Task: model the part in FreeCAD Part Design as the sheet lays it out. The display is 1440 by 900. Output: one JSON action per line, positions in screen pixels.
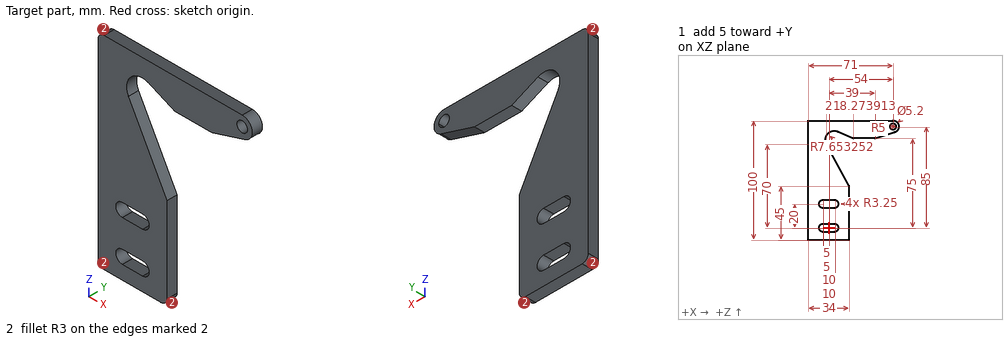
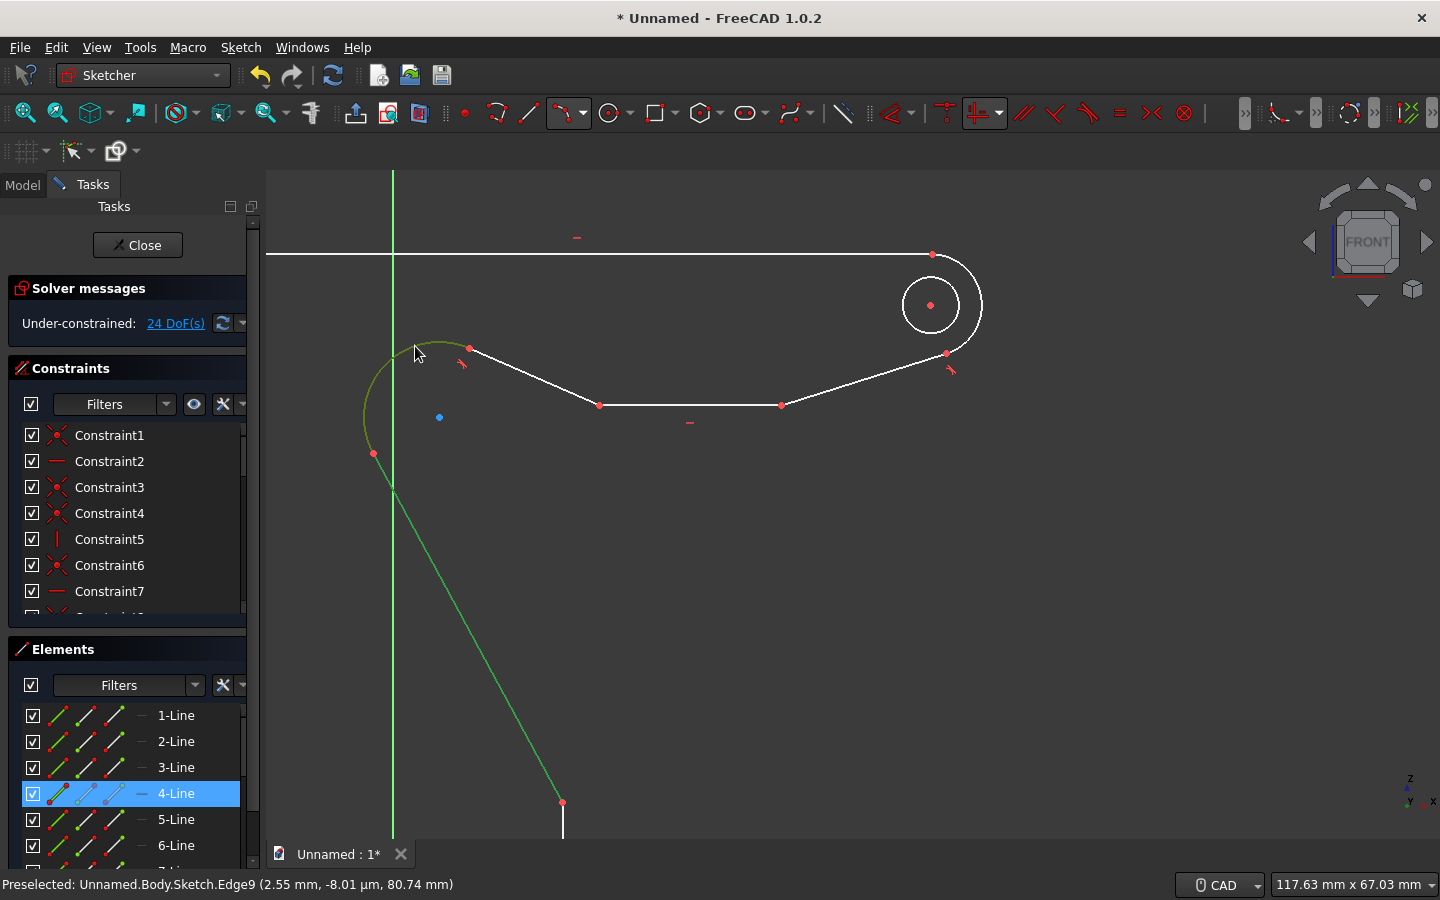
{"action": "left_click", "coordinate": [1088, 114]}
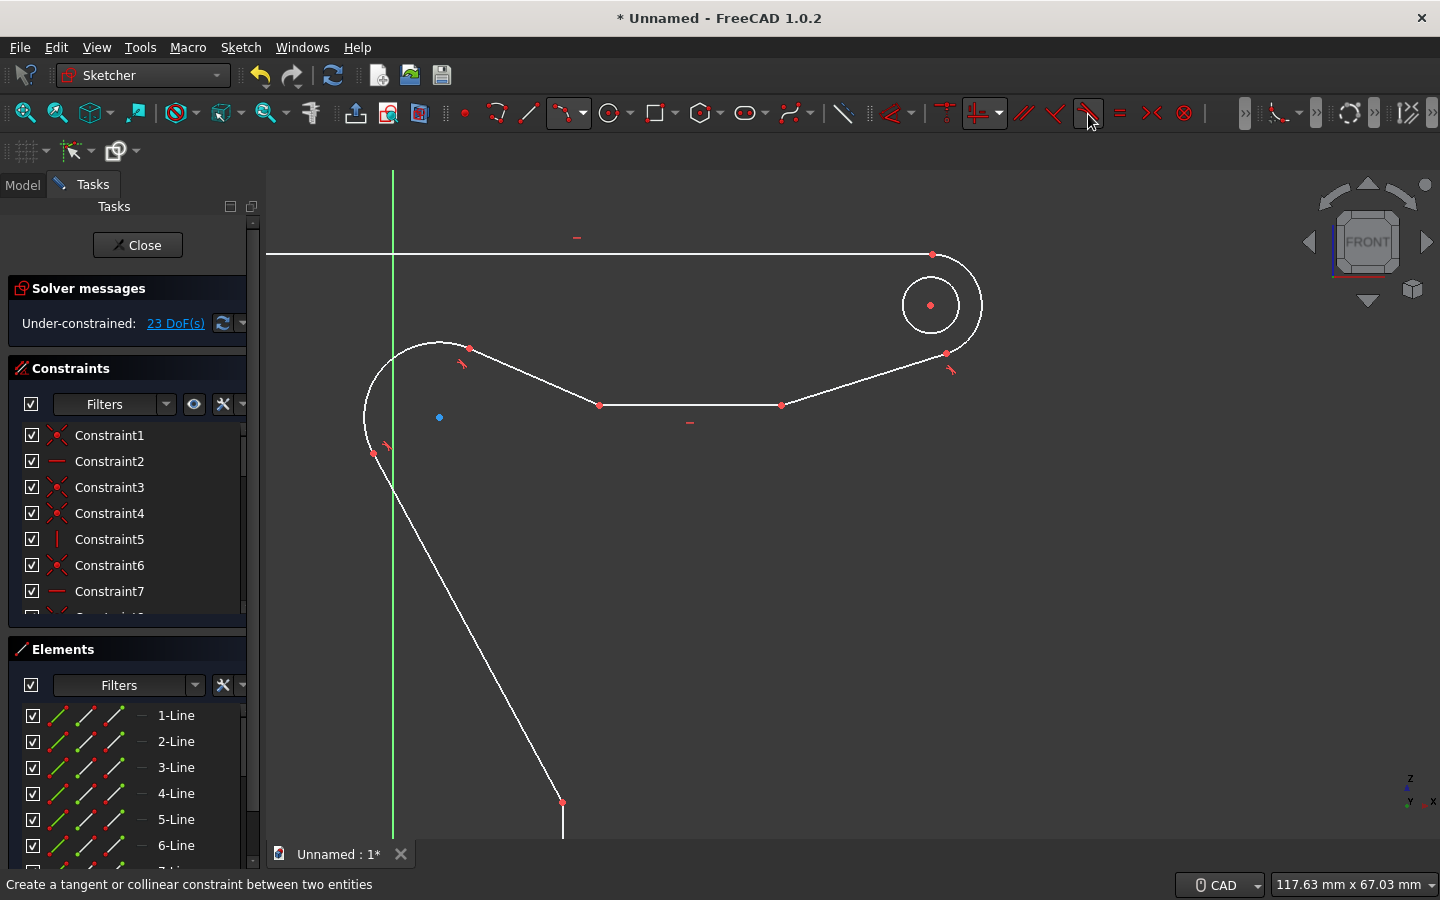
{"action": "left_click", "coordinate": [435, 254]}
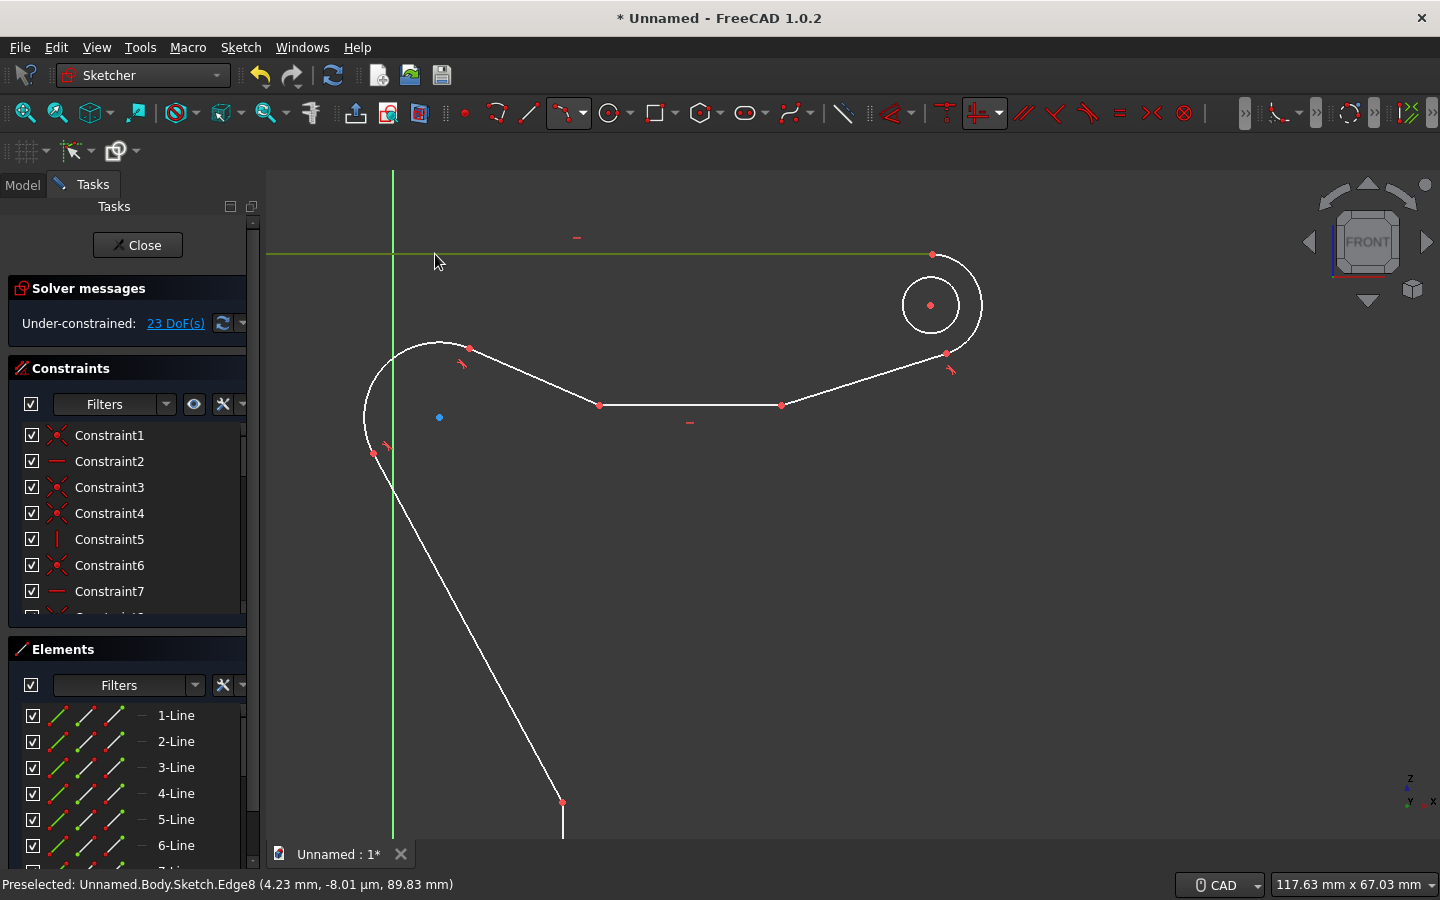
{"action": "left_click", "coordinate": [977, 326]}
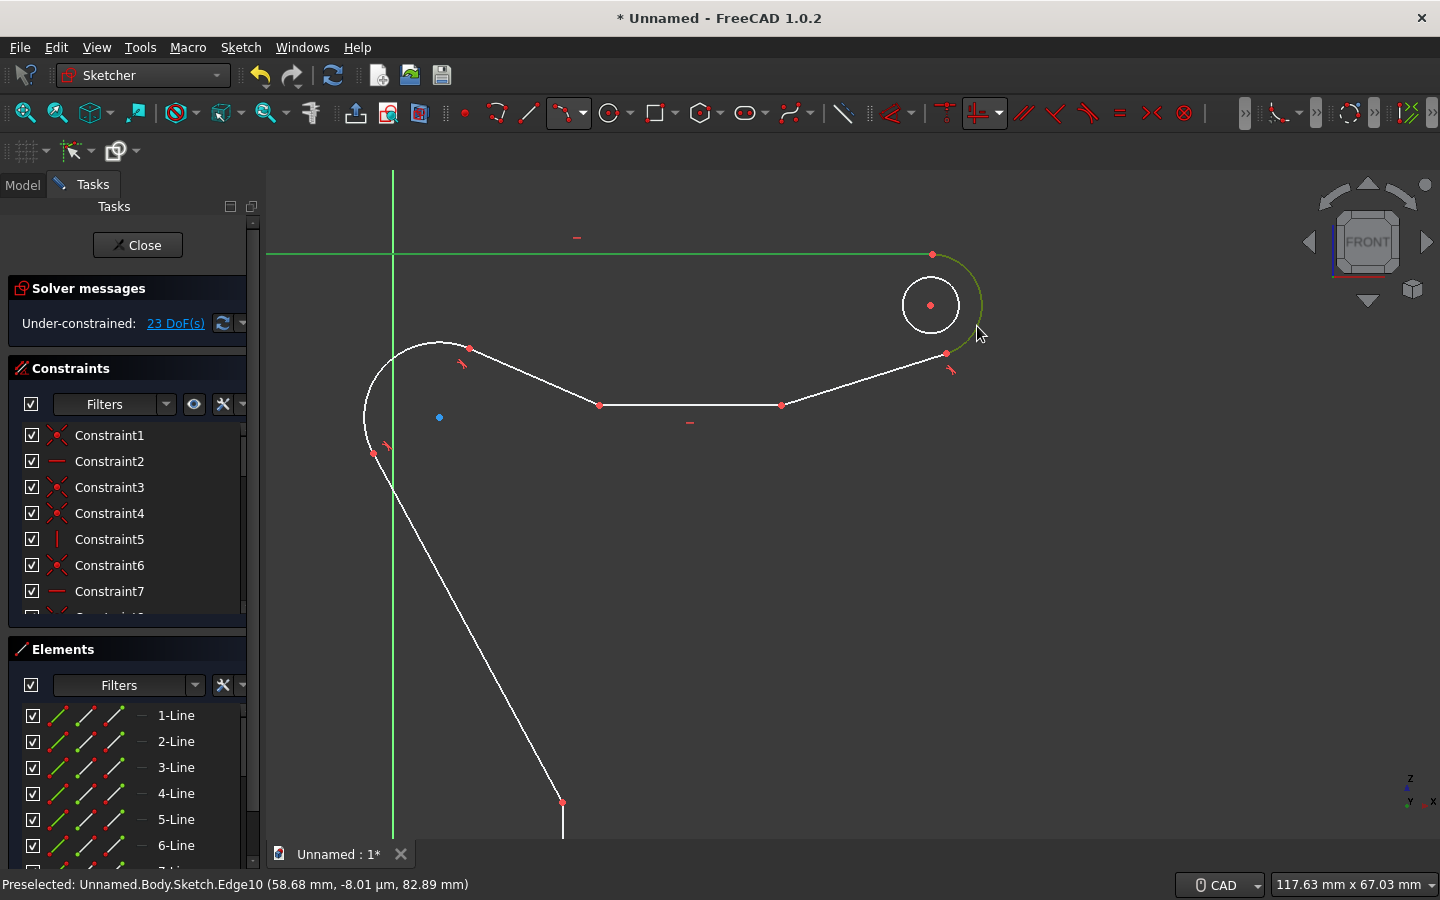
{"action": "left_click", "coordinate": [1088, 114]}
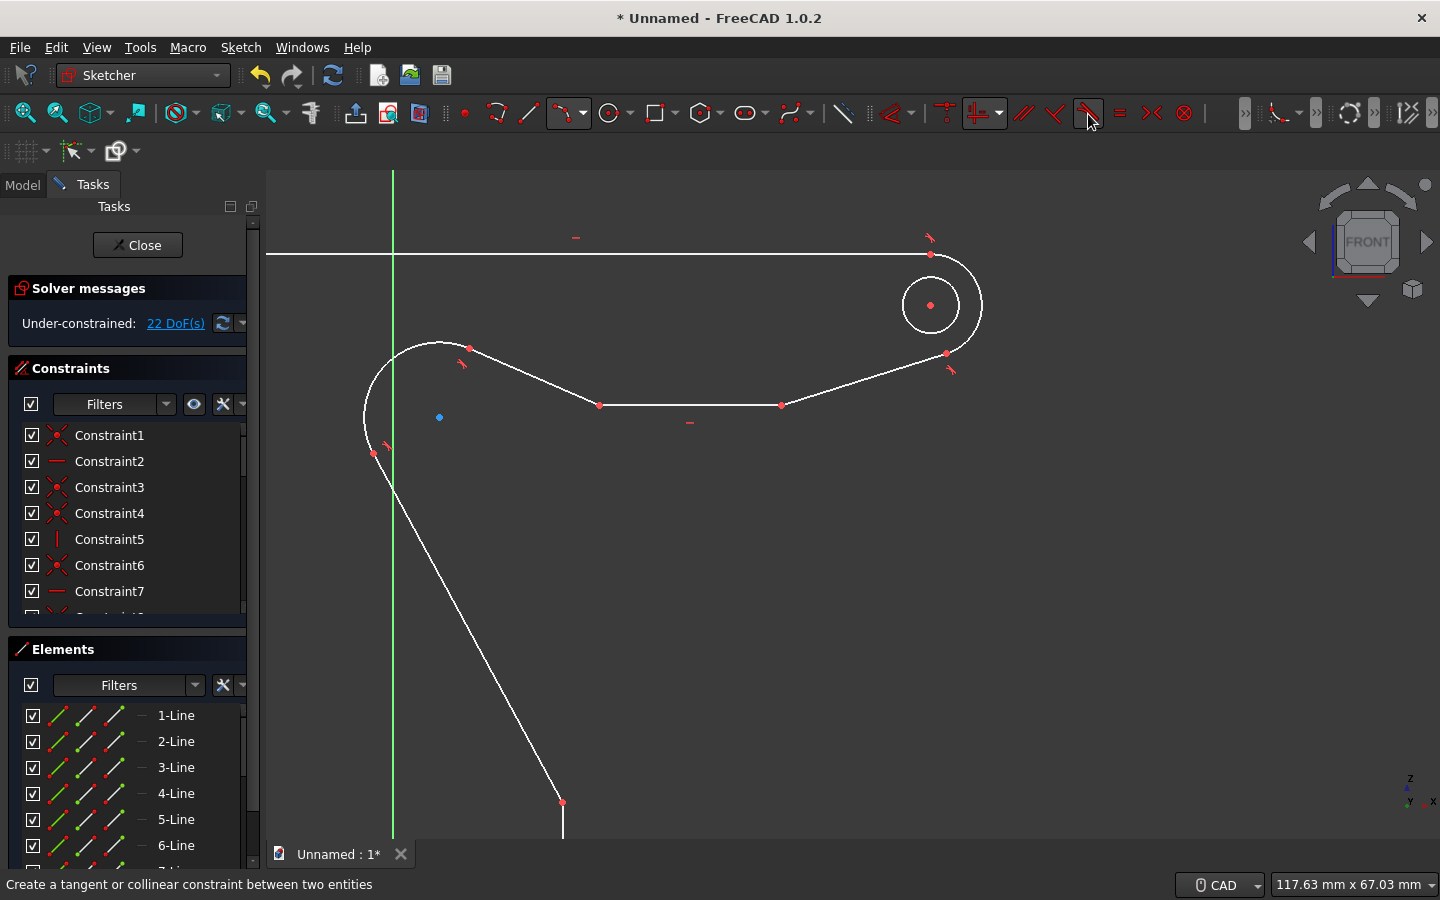
{"action": "scroll", "coordinate": [933, 303], "scroll_direction": "down", "scroll_amount": 4}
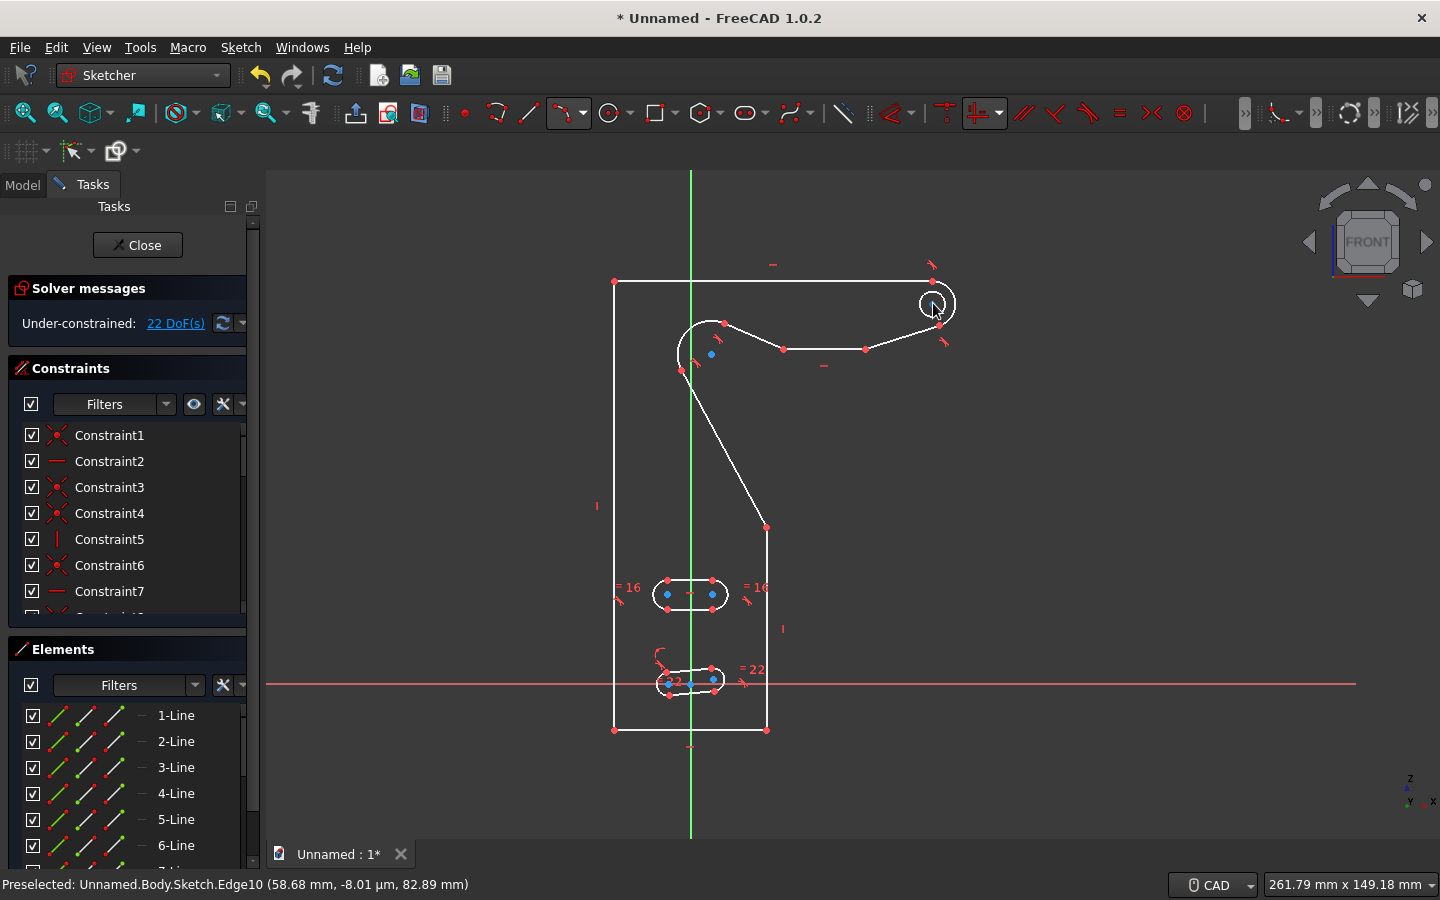
{"action": "scroll", "coordinate": [680, 671], "scroll_direction": "up", "scroll_amount": 2}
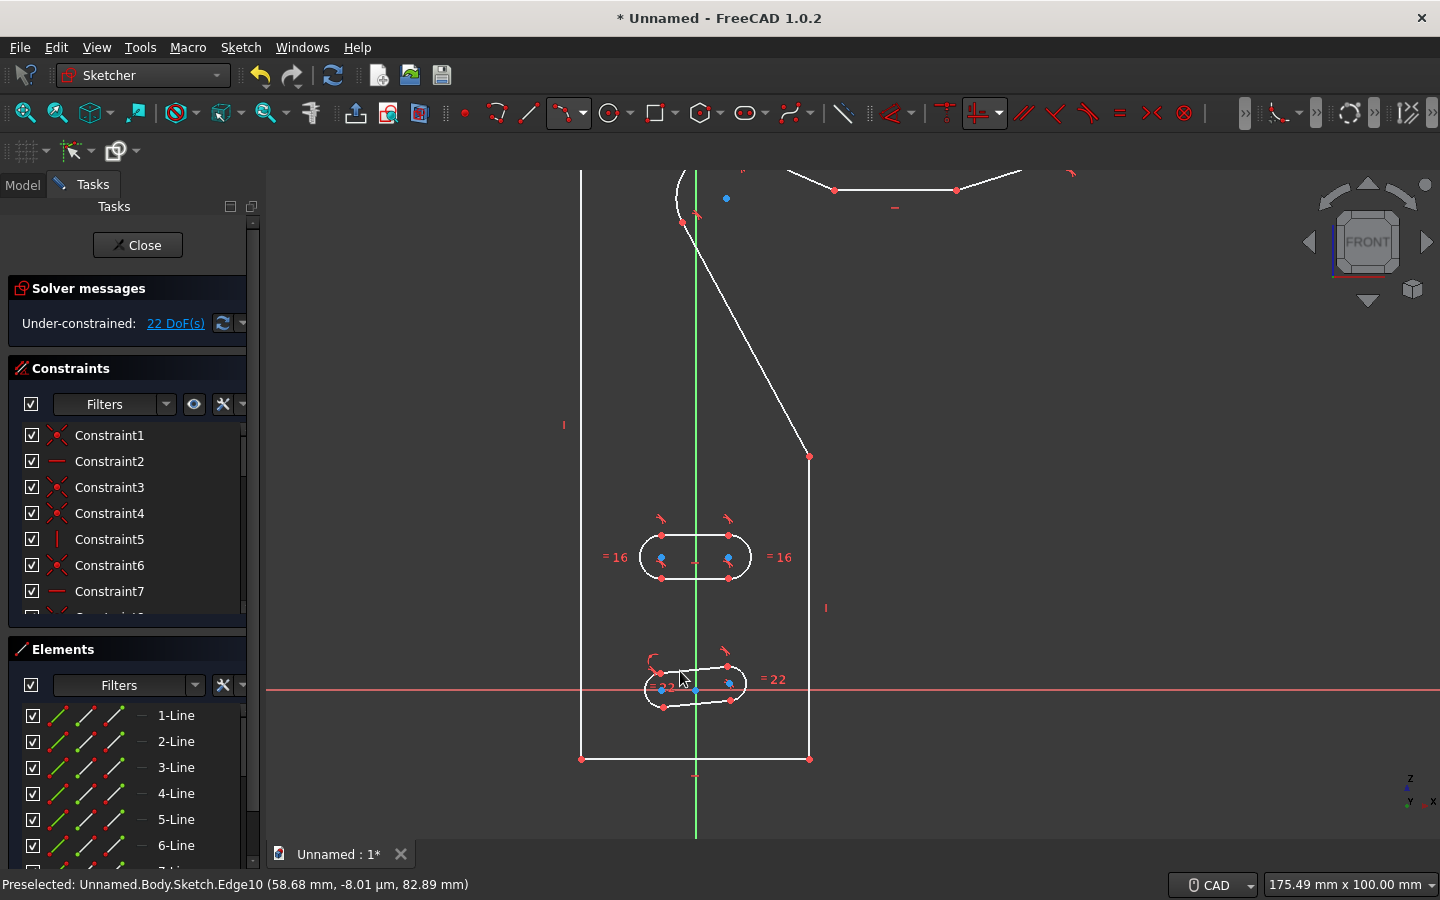
{"action": "left_click", "coordinate": [681, 671]}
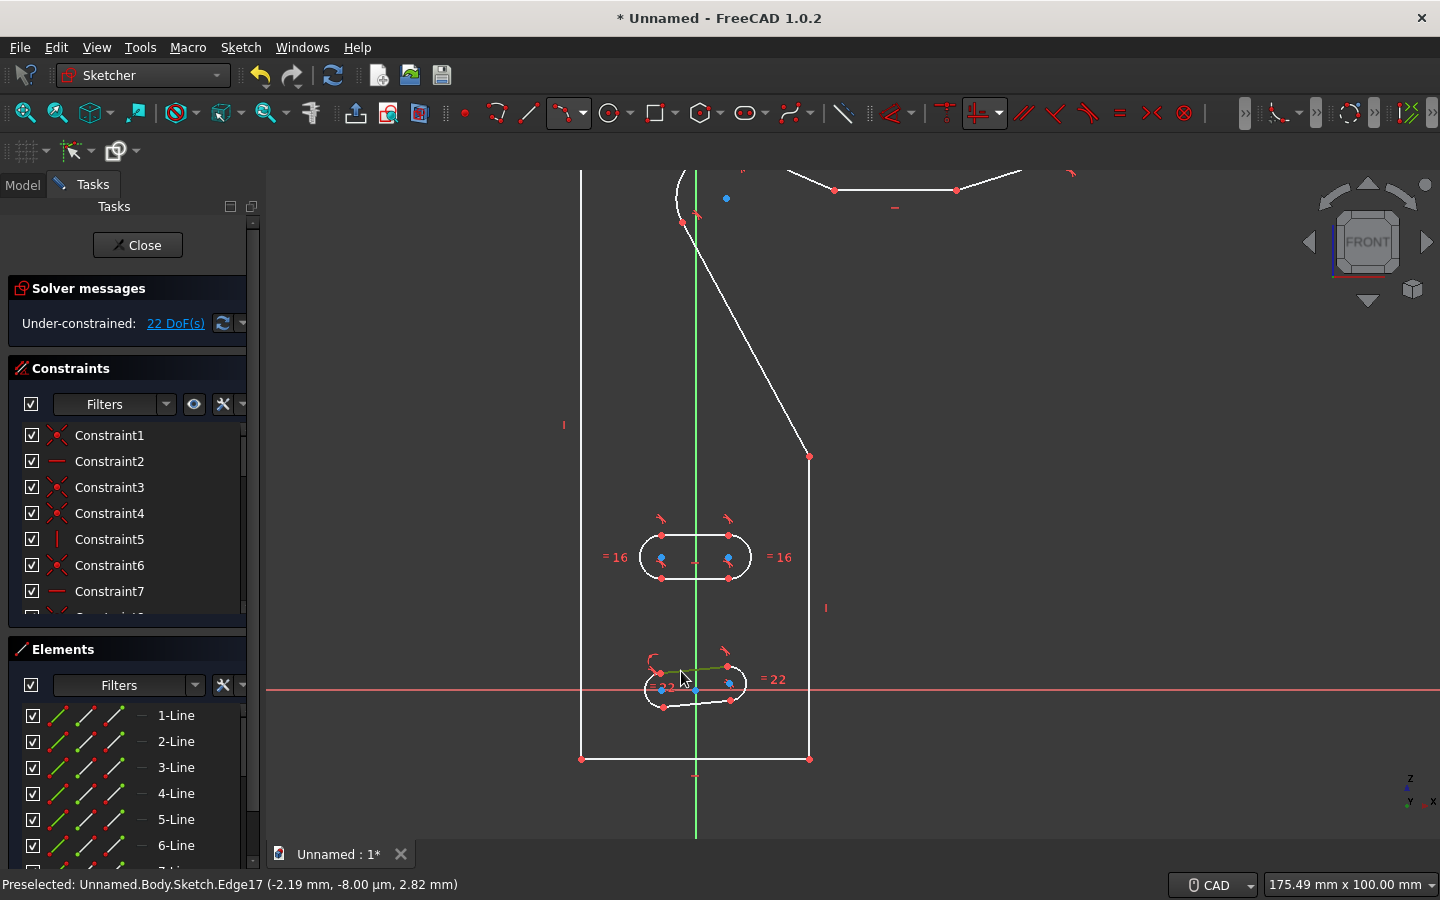
{"action": "left_click", "coordinate": [1002, 114]}